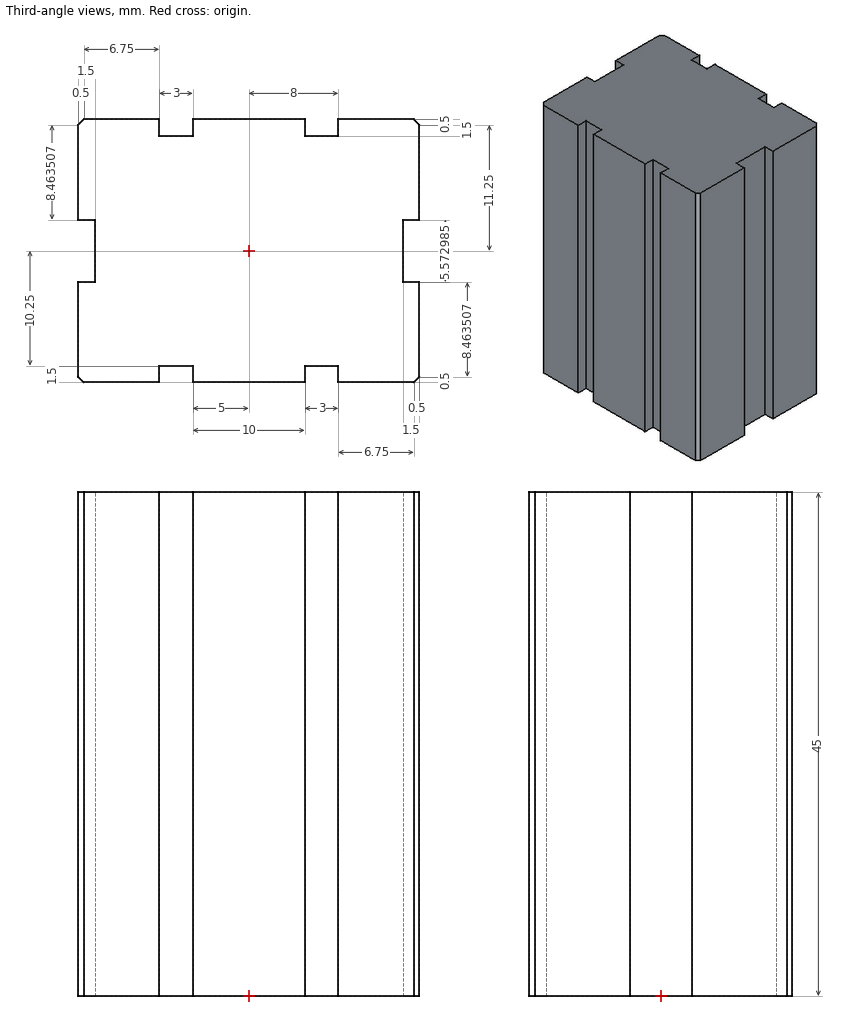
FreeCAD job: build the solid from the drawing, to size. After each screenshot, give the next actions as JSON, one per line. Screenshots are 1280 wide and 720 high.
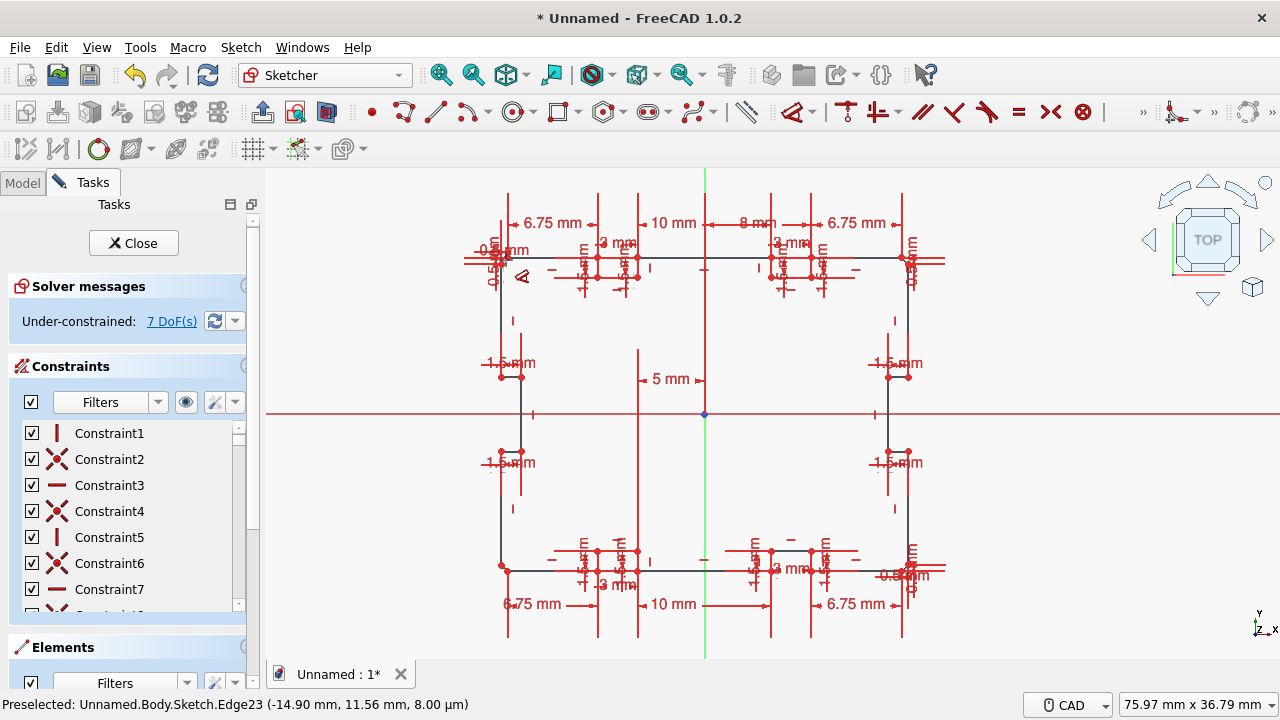
{"action": "scroll", "coordinate": [503, 567], "scroll_direction": "up", "scroll_amount": 9}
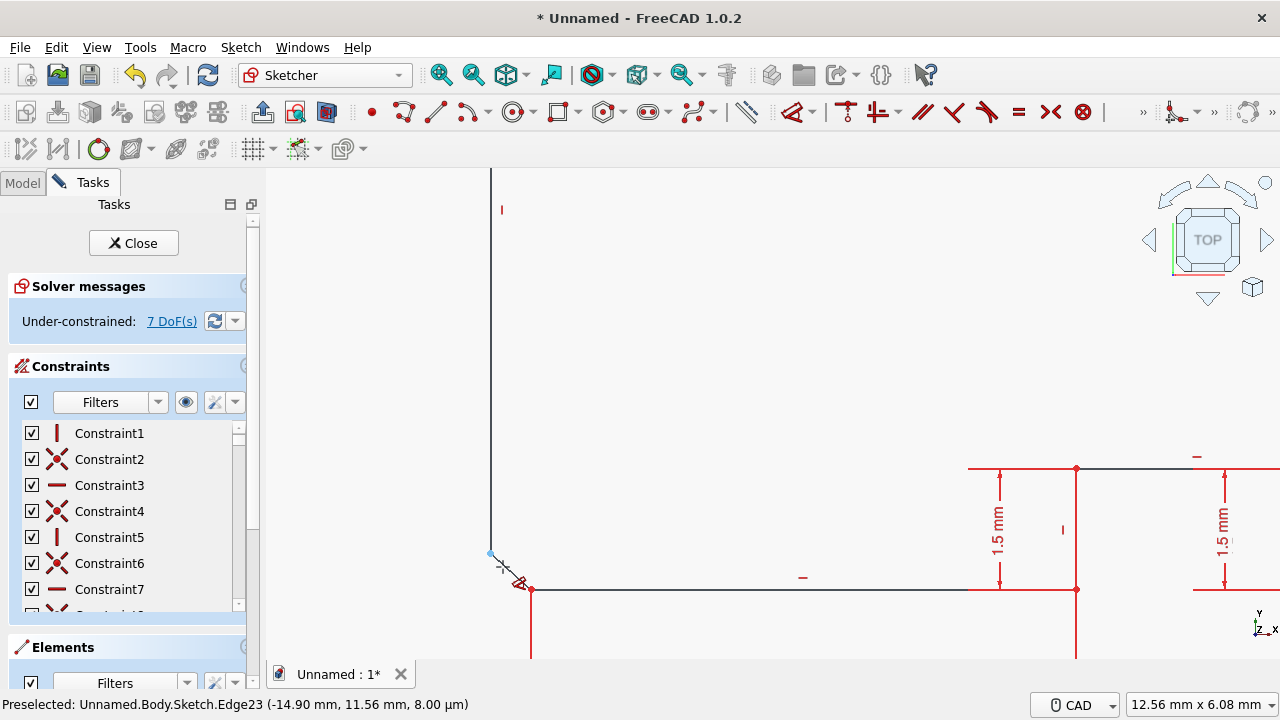
{"action": "left_click", "coordinate": [503, 564]}
{"action": "left_click", "coordinate": [457, 572]}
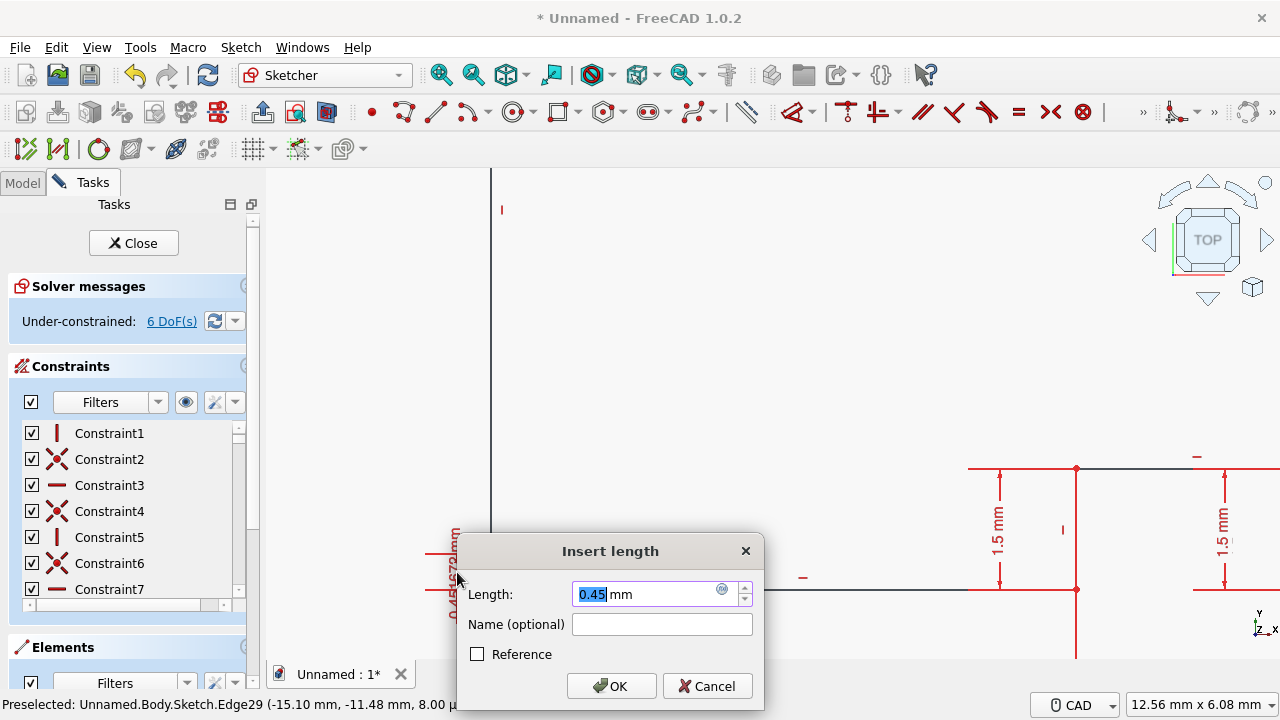
{"action": "type", "text": "0.5"}
{"action": "key", "text": "Return"}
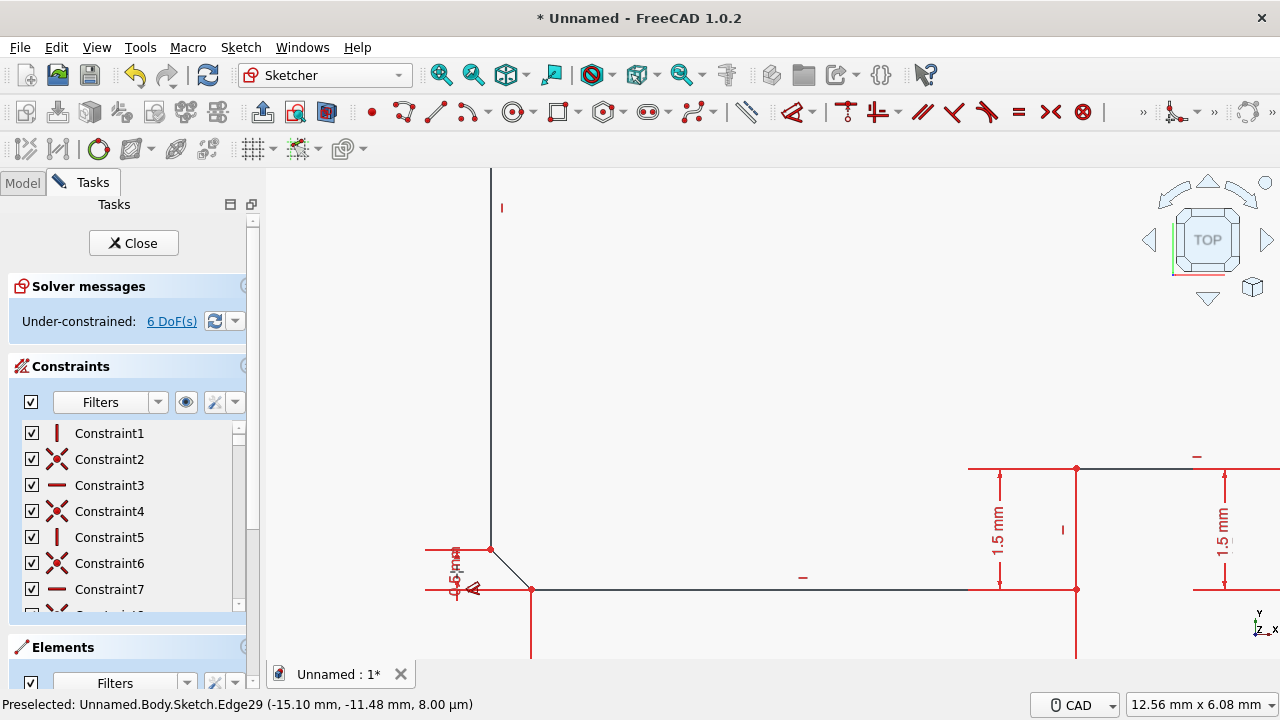
{"action": "scroll", "coordinate": [503, 567], "scroll_direction": "down", "scroll_amount": 9}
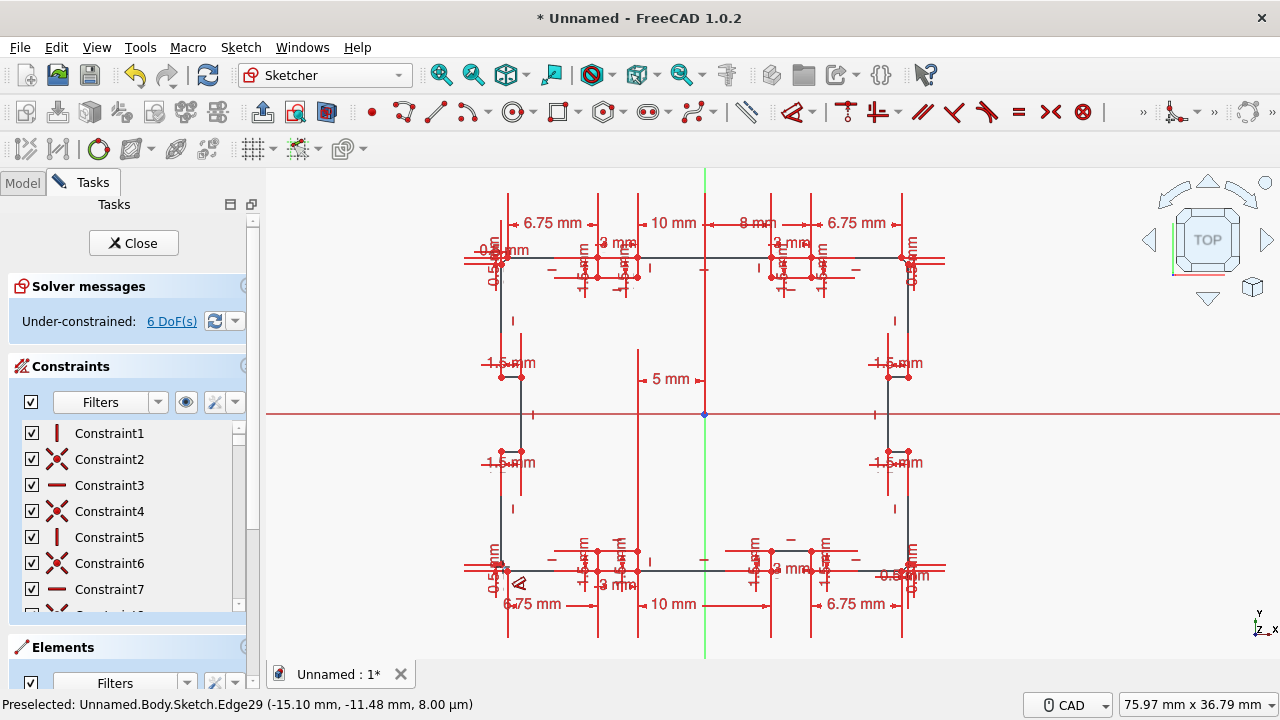
{"action": "left_click", "coordinate": [638, 551]}
{"action": "left_click", "coordinate": [604, 483]}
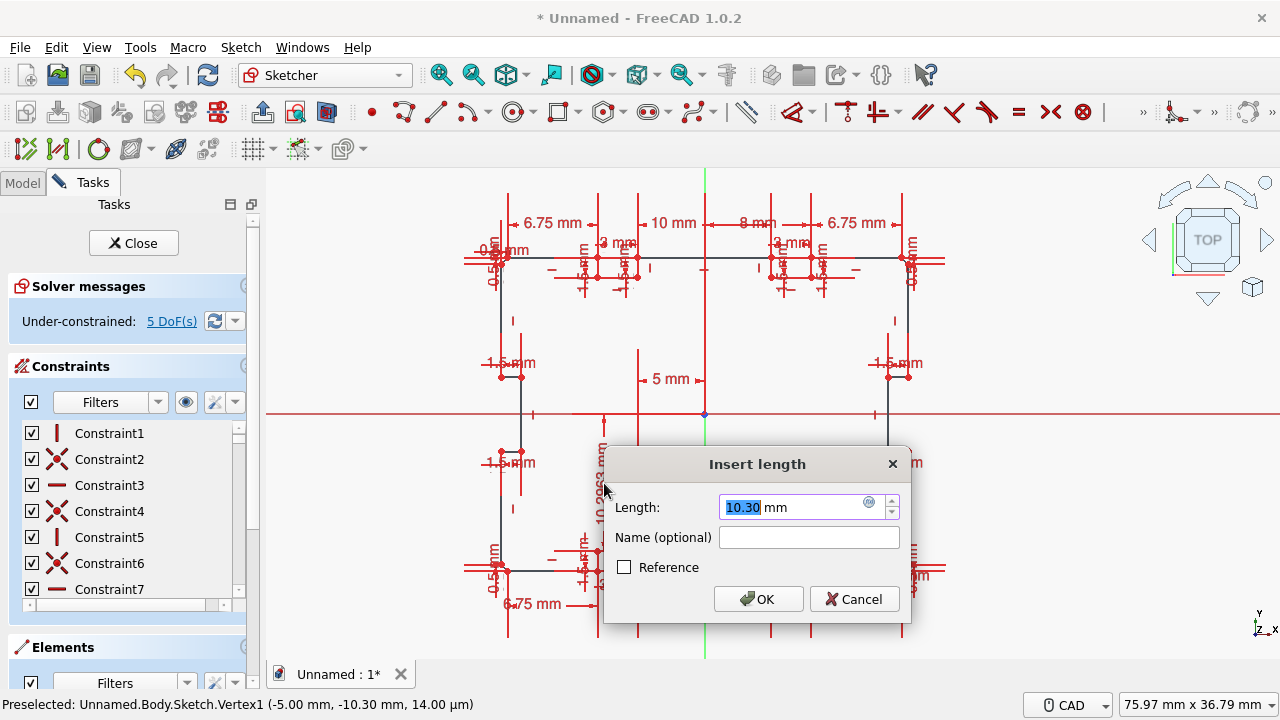
{"action": "type", "text": "10.25"}
{"action": "key", "text": "Return"}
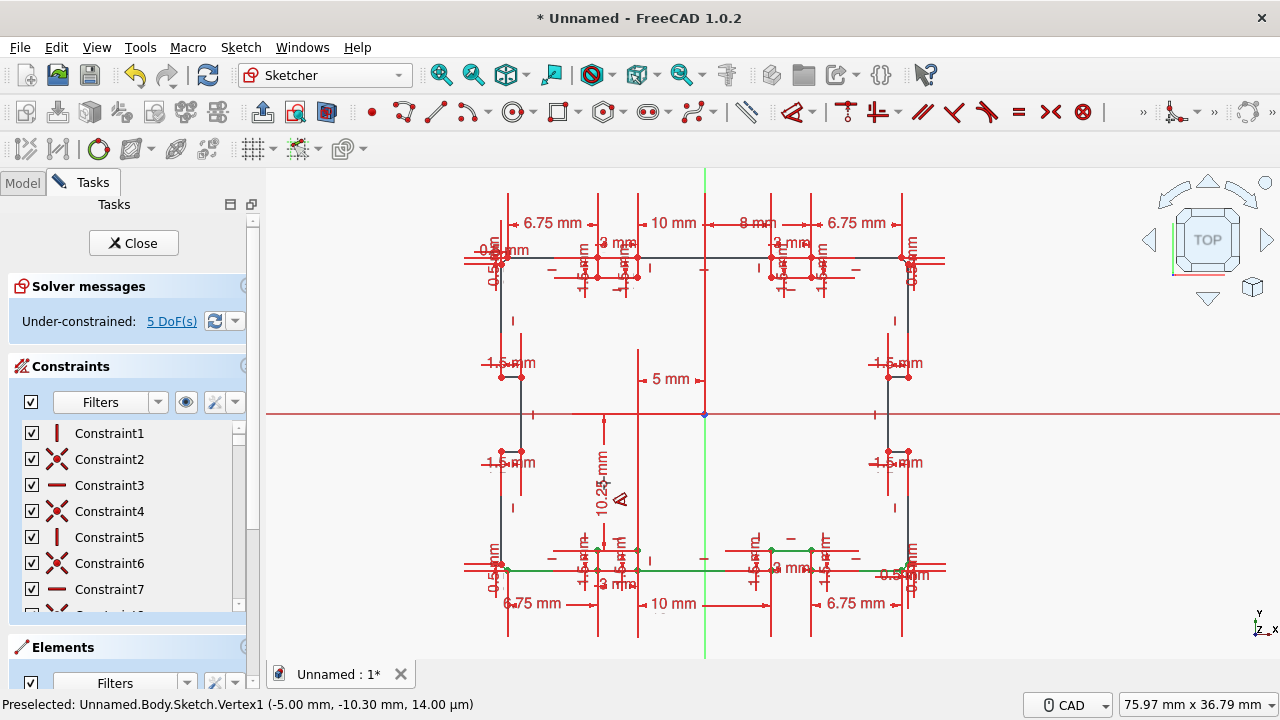
{"action": "scroll", "coordinate": [908, 264], "scroll_direction": "up", "scroll_amount": 2}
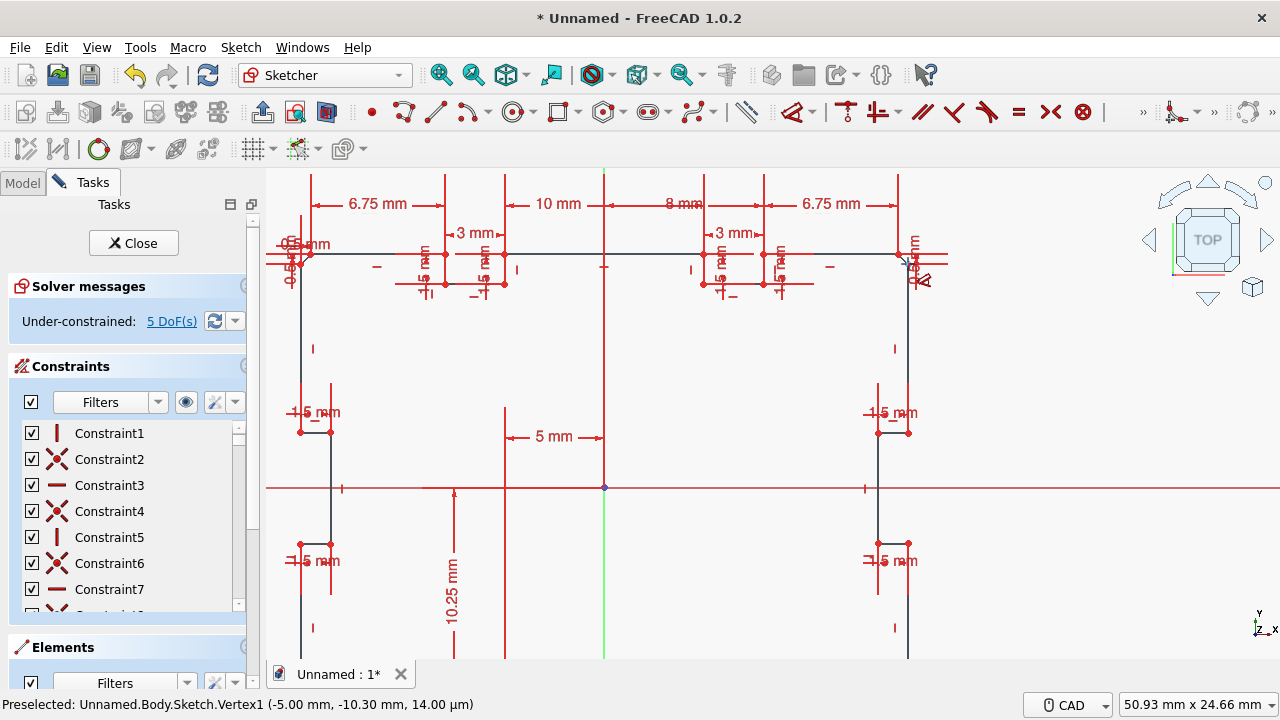
{"action": "left_click", "coordinate": [908, 264]}
{"action": "left_click", "coordinate": [942, 376]}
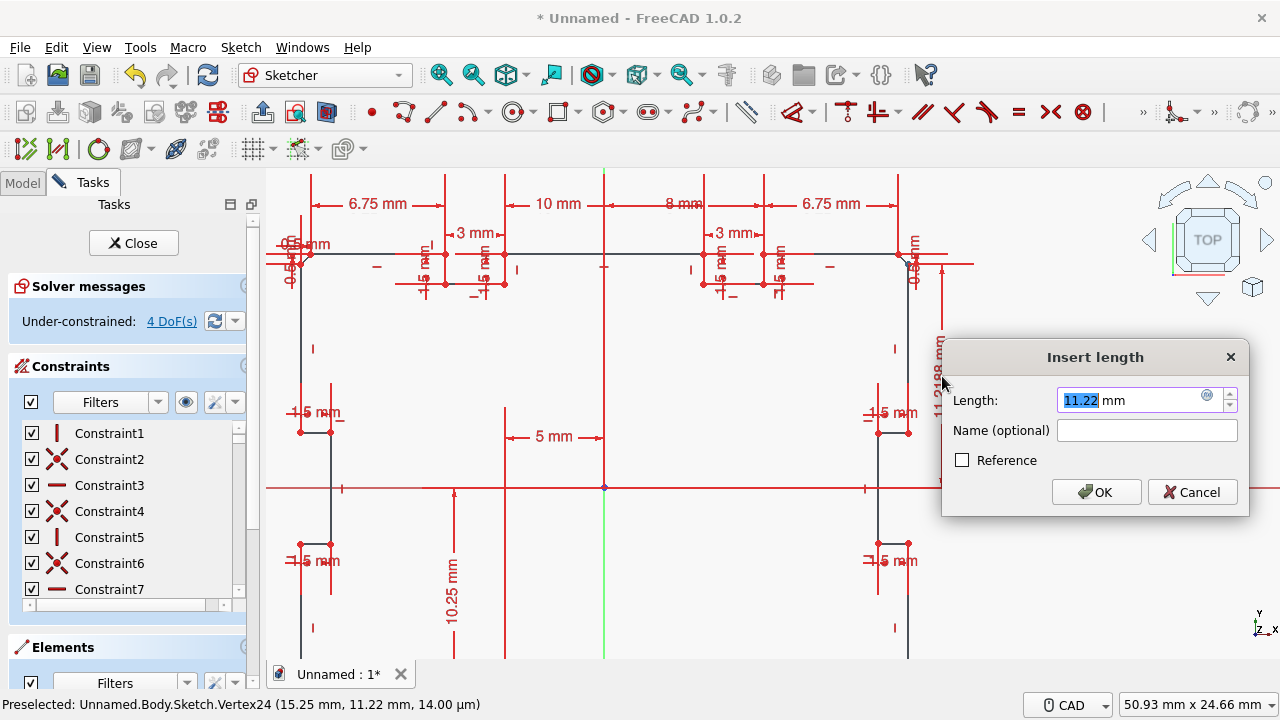
{"action": "type", "text": "11.25"}
{"action": "key", "text": "Return"}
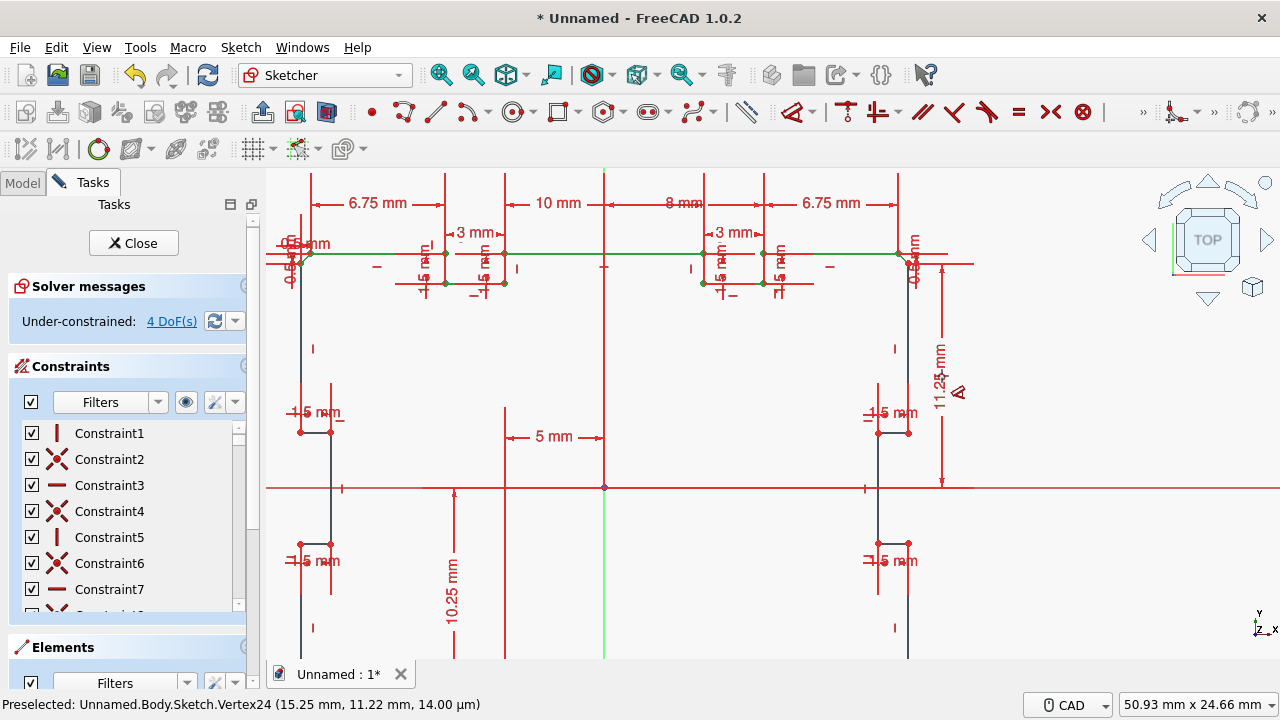
{"action": "left_click", "coordinate": [908, 594]}
{"action": "left_click", "coordinate": [942, 587]}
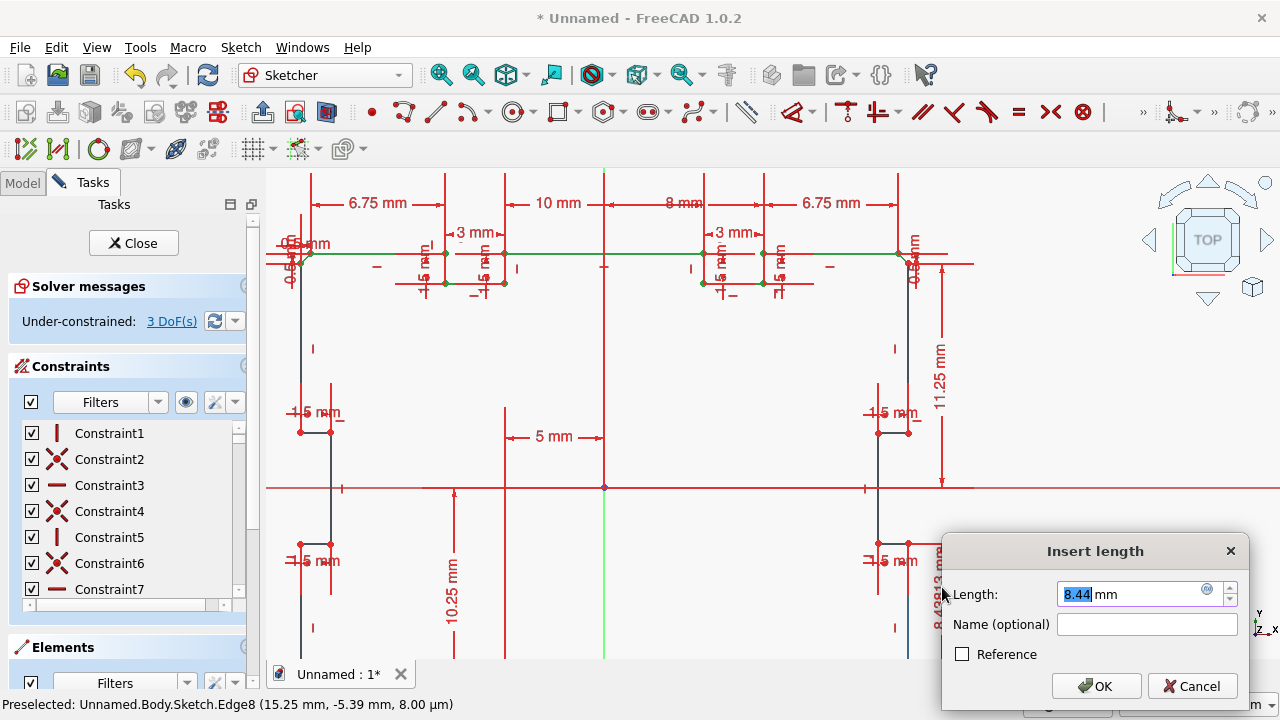
{"action": "type", "text": "8.463507"}
{"action": "key", "text": "Return"}